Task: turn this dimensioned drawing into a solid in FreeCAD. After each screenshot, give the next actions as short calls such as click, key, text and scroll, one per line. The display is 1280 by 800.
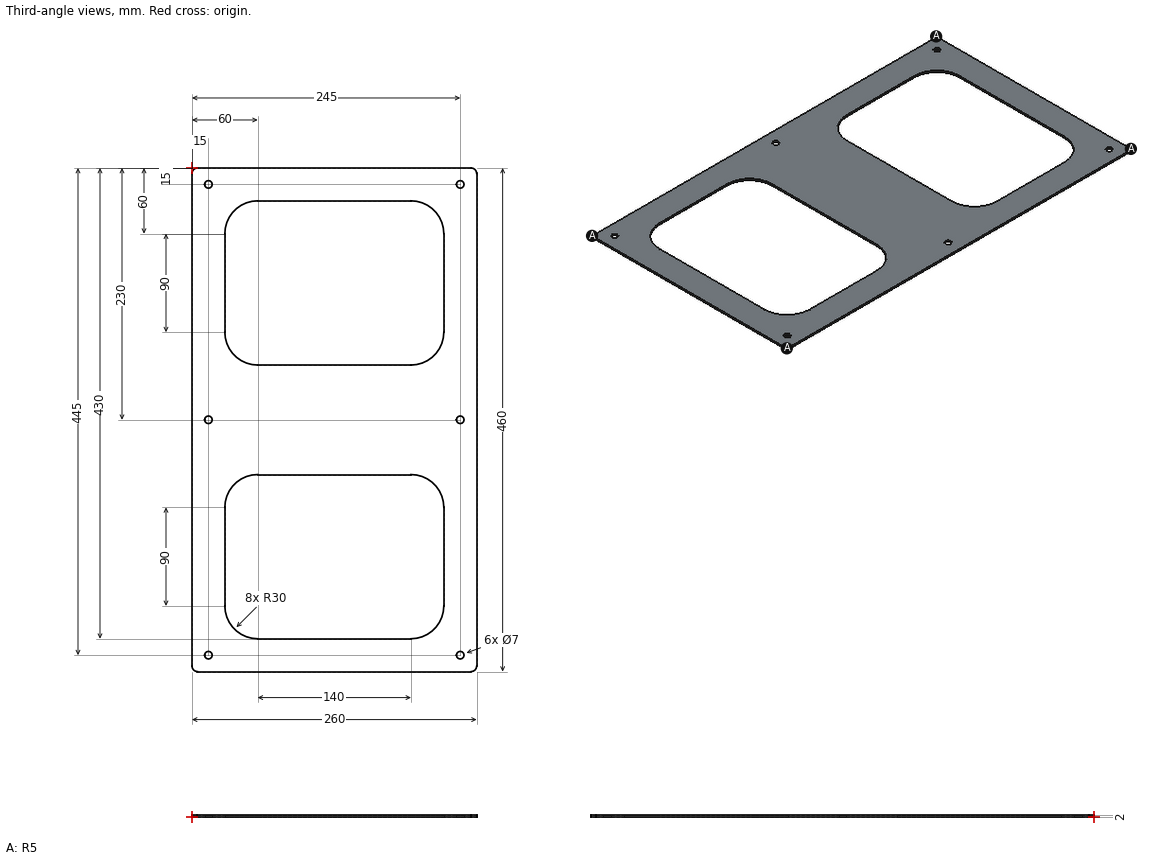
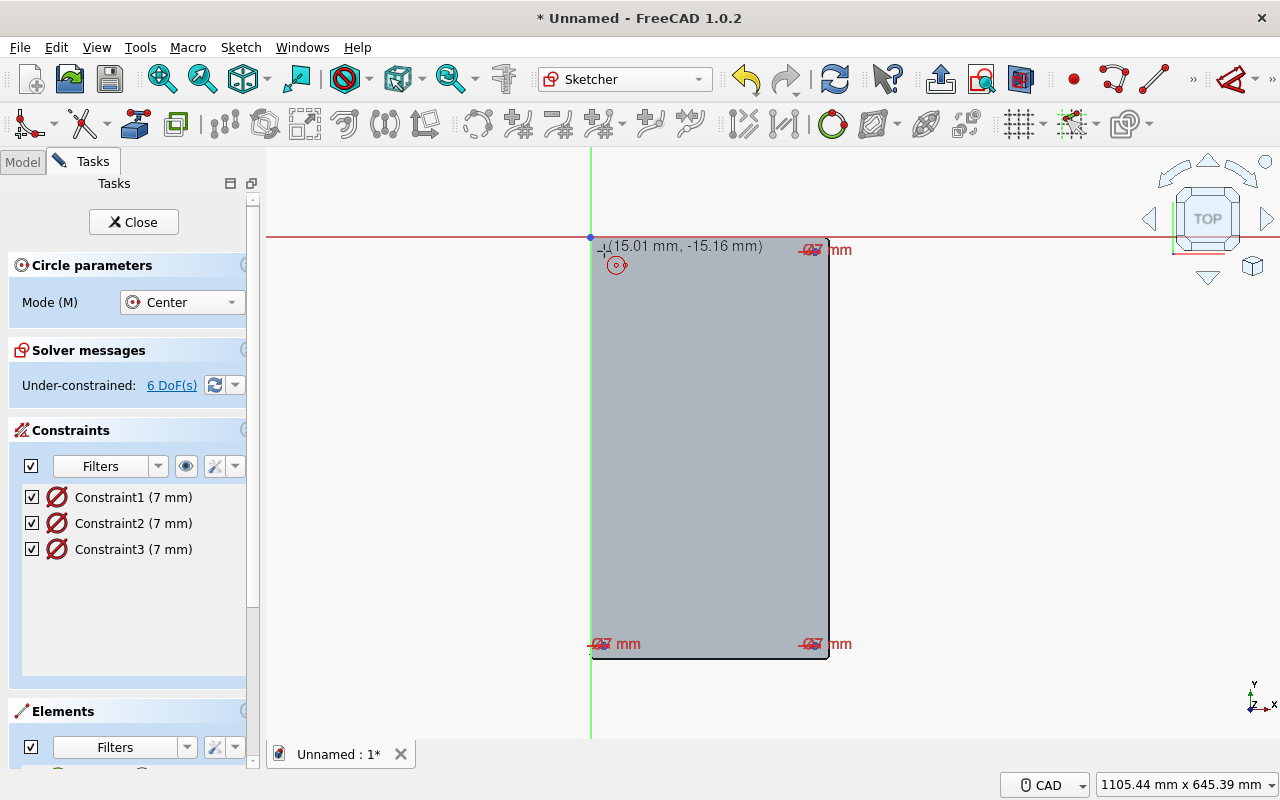
click(604, 251)
move(607, 253)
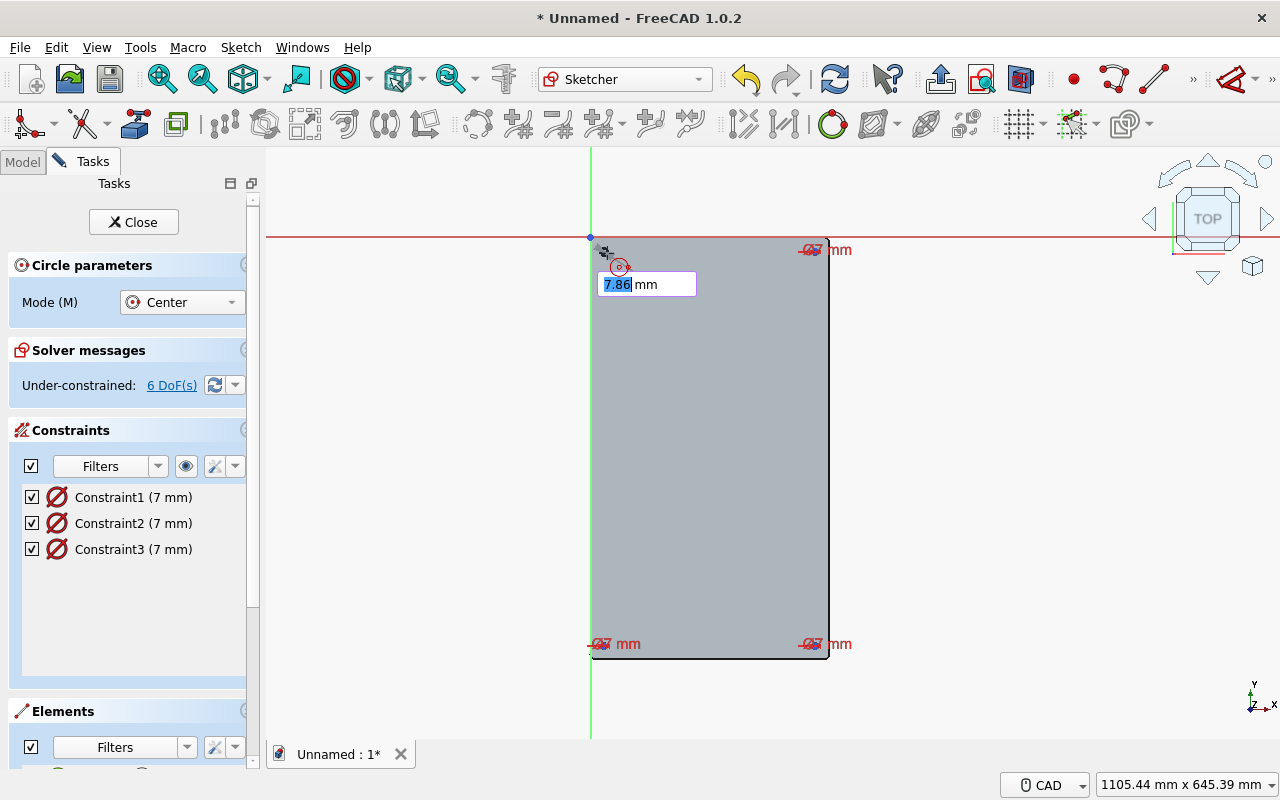
text(7)
key(Return)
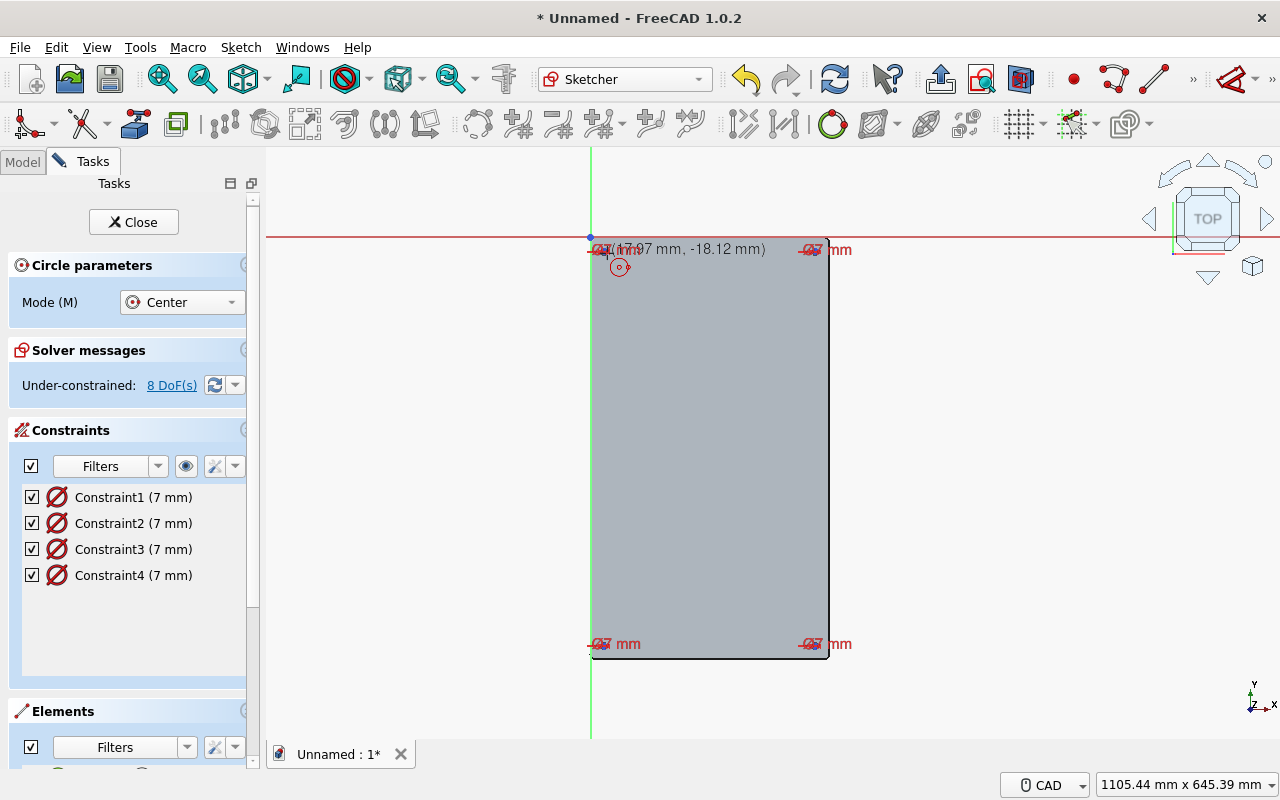
scroll(815, 448, up, 10)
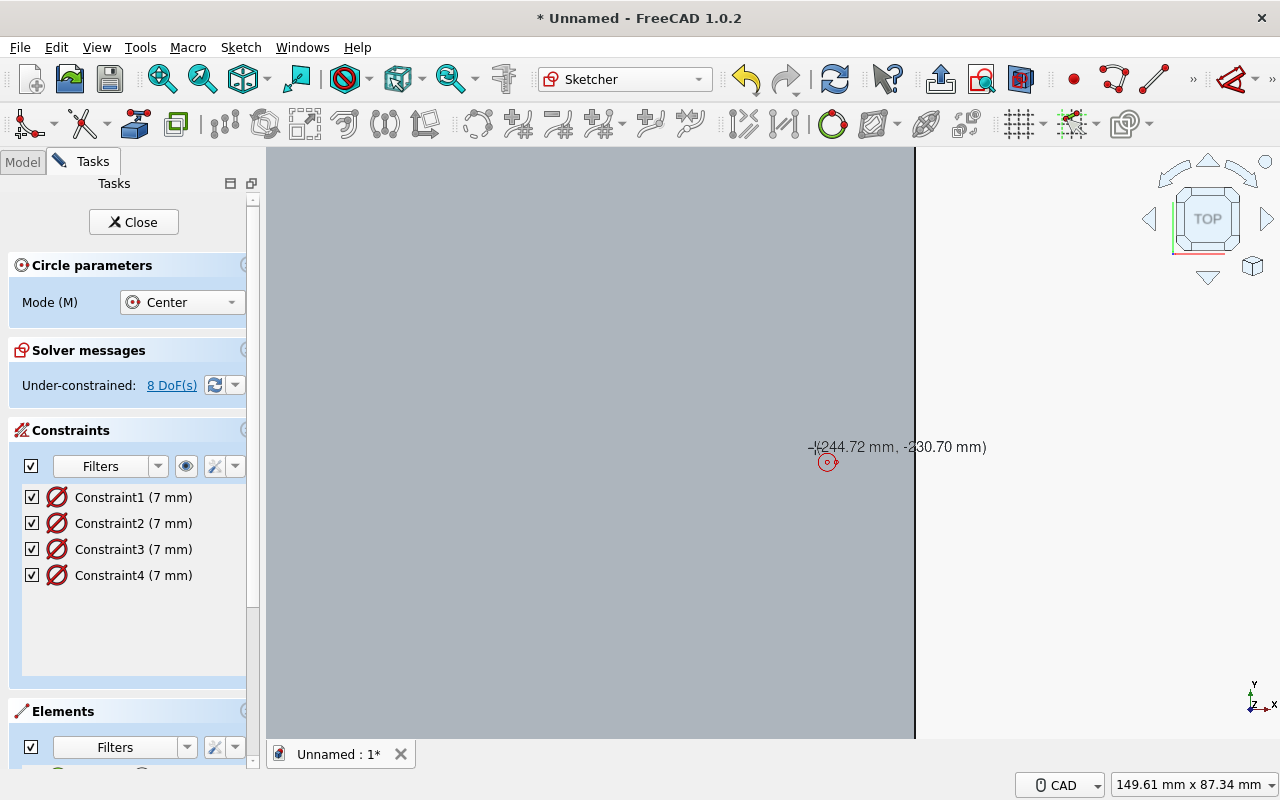
scroll(816, 448, down, 10)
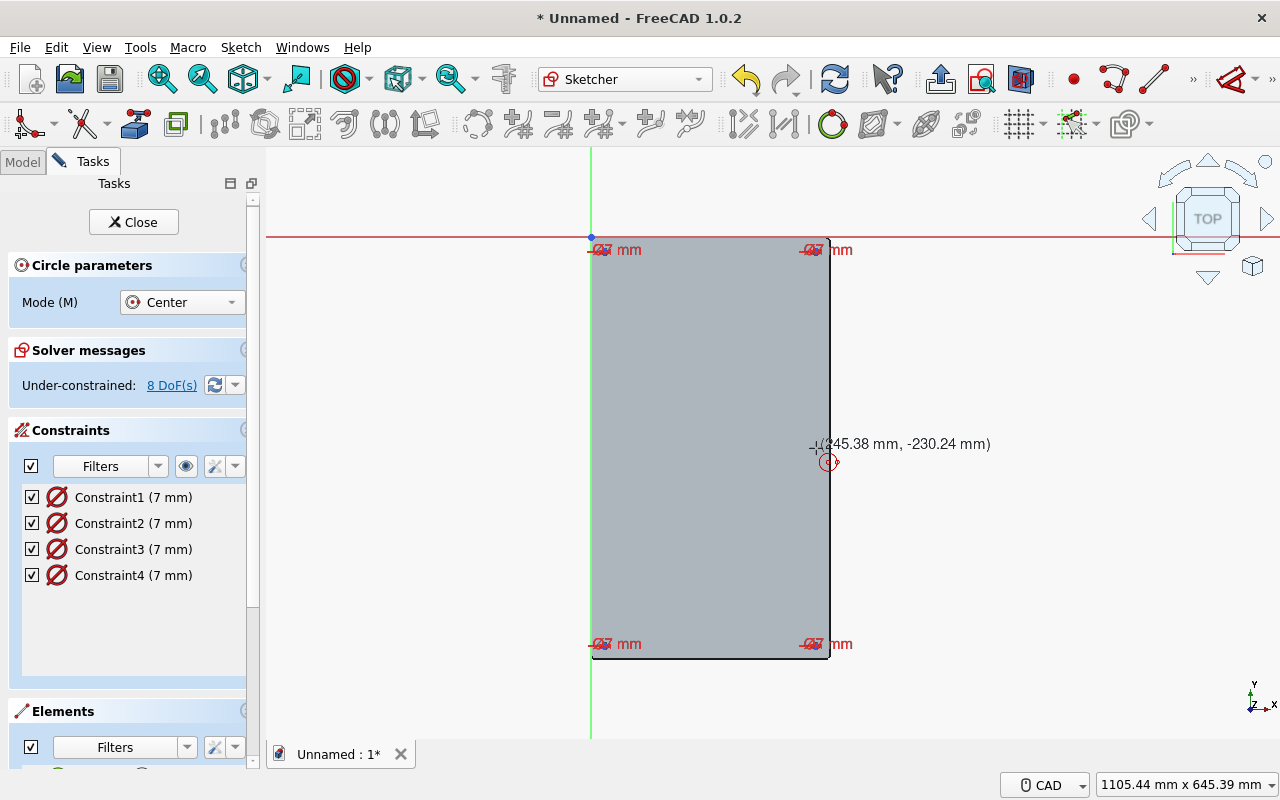
click(816, 448)
move(818, 446)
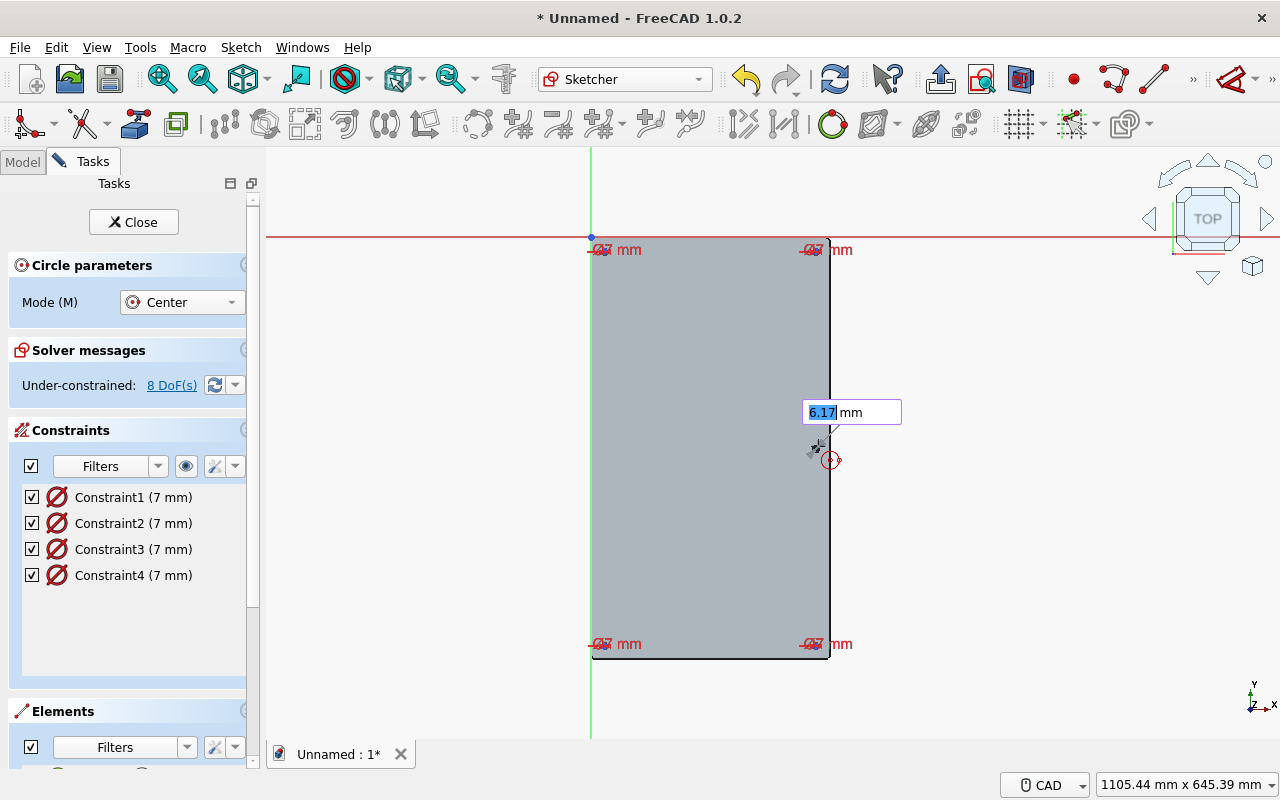
text(7)
key(Return)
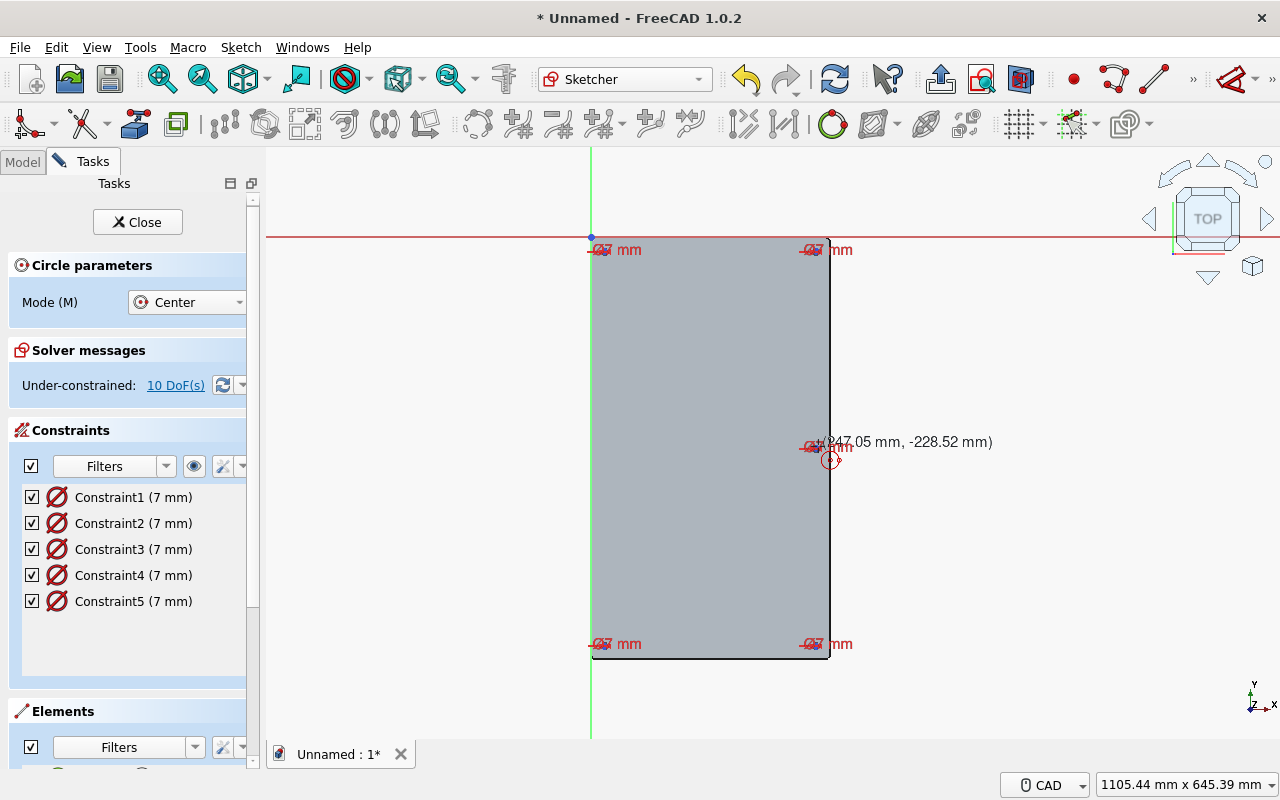
scroll(605, 448, up, 10)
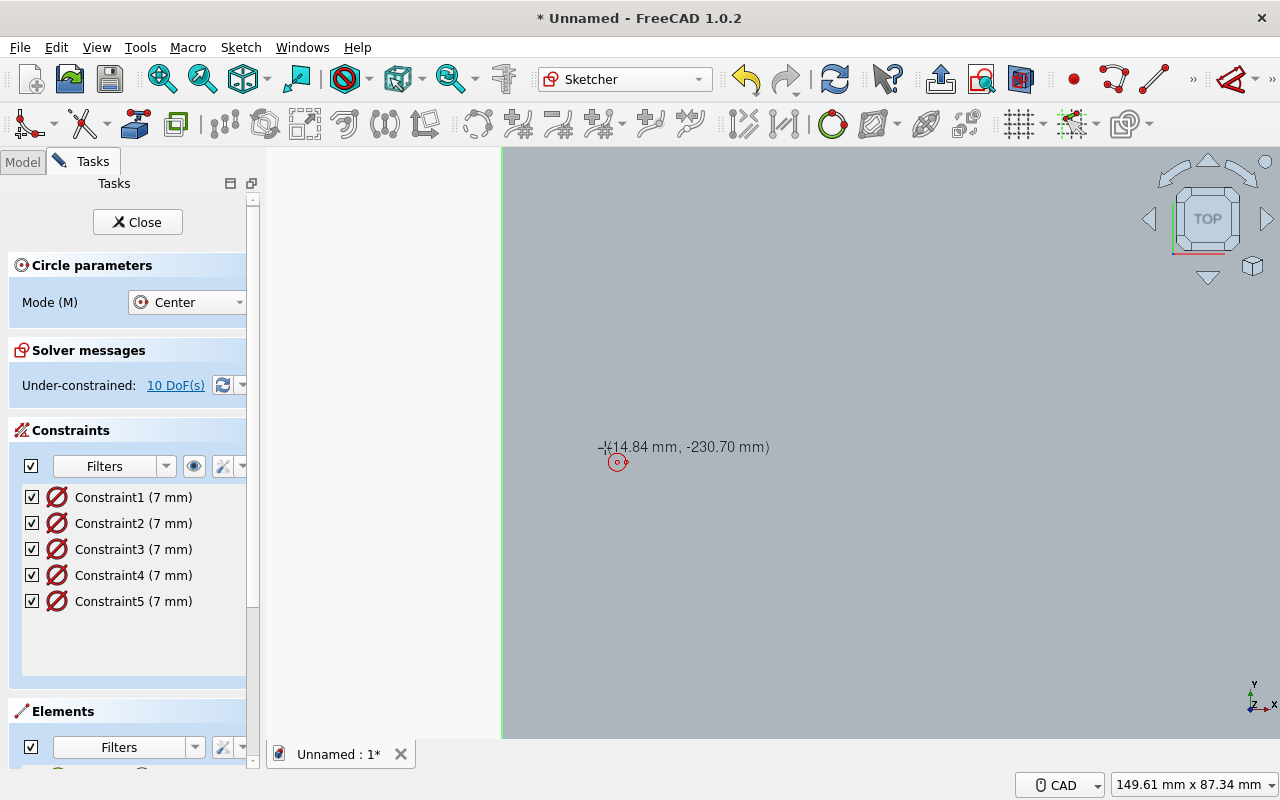
scroll(604, 448, down, 10)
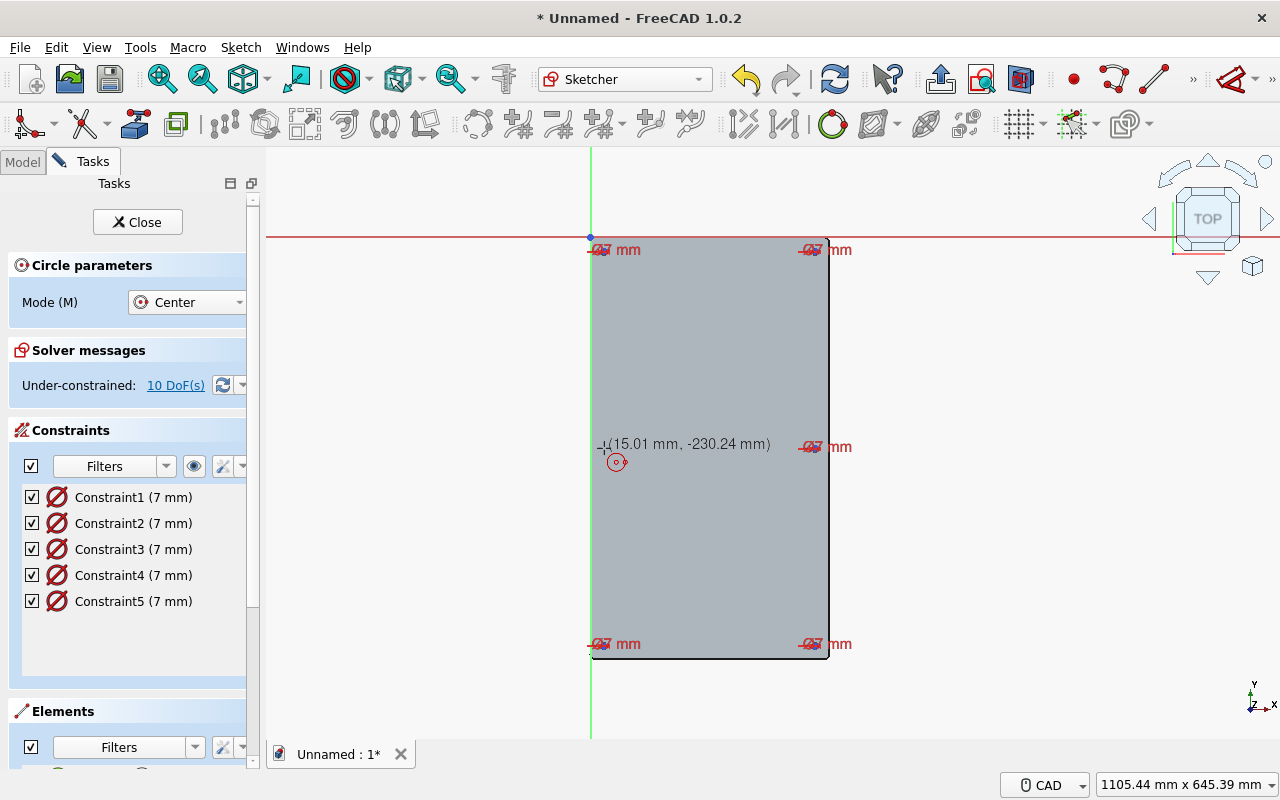
click(604, 448)
move(607, 446)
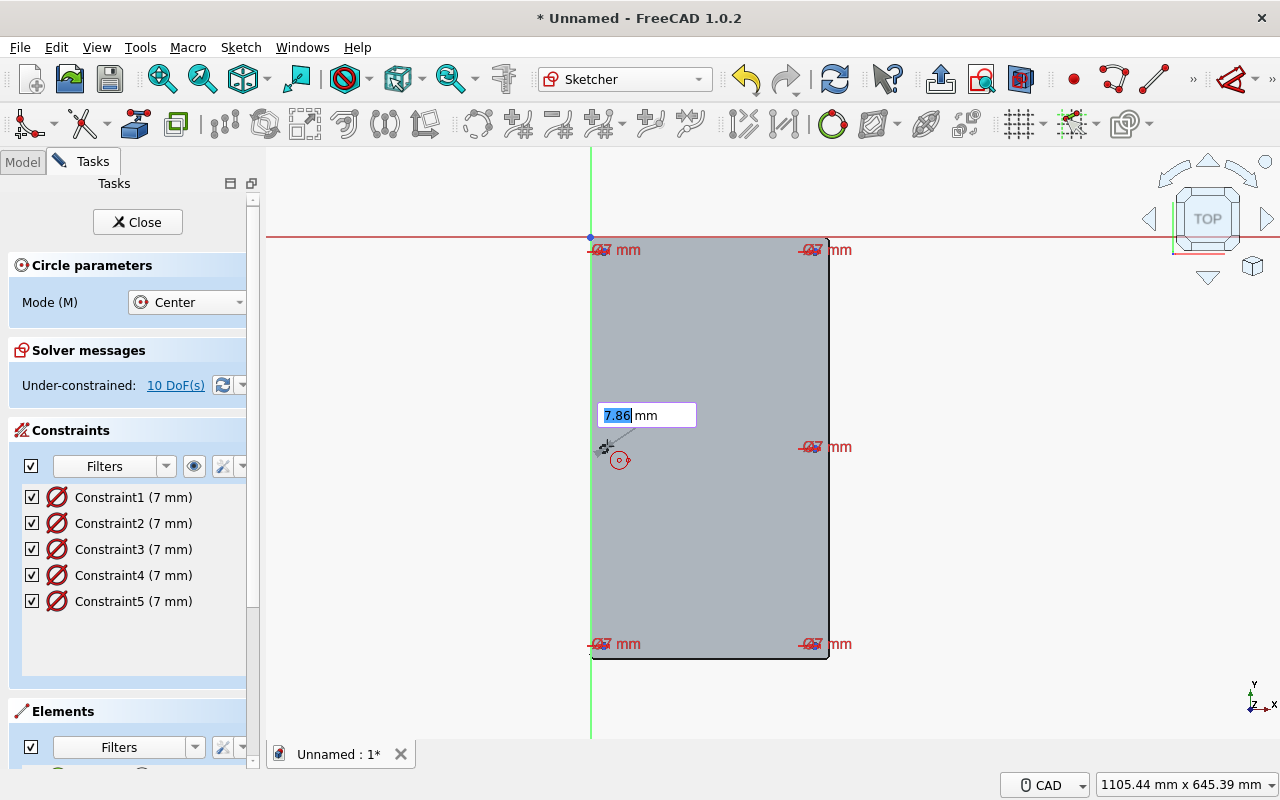
text(7)
key(Return)
key(Escape)